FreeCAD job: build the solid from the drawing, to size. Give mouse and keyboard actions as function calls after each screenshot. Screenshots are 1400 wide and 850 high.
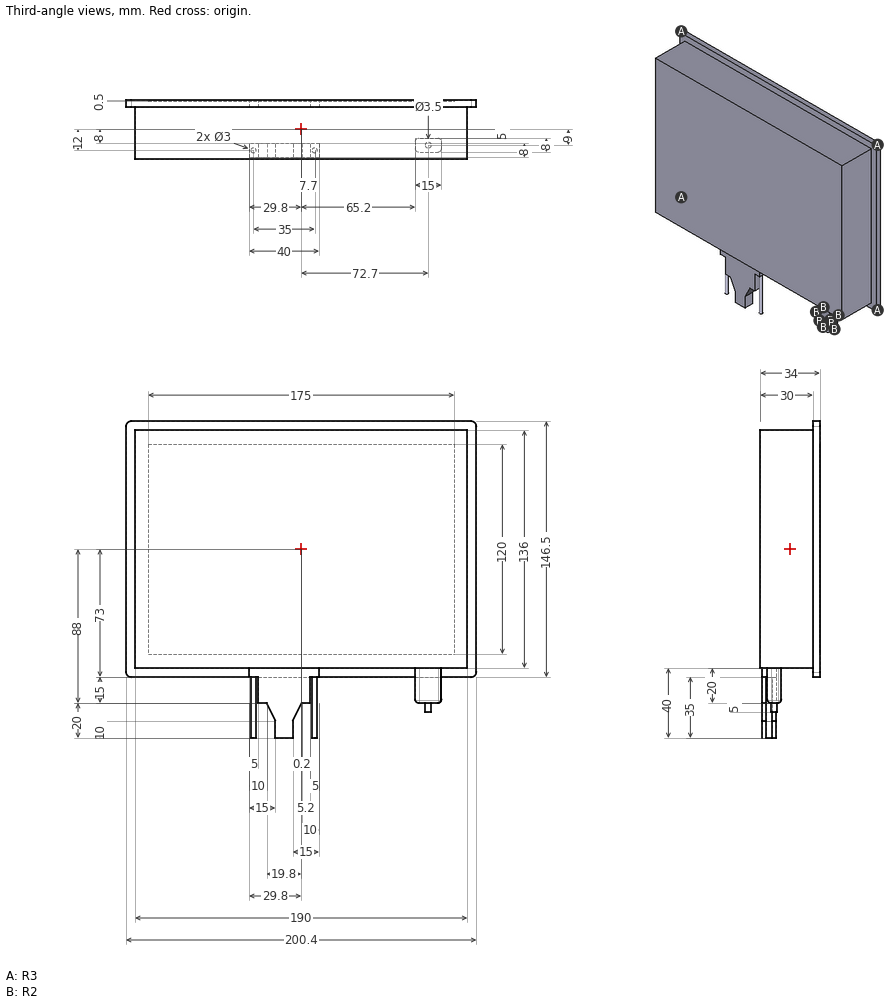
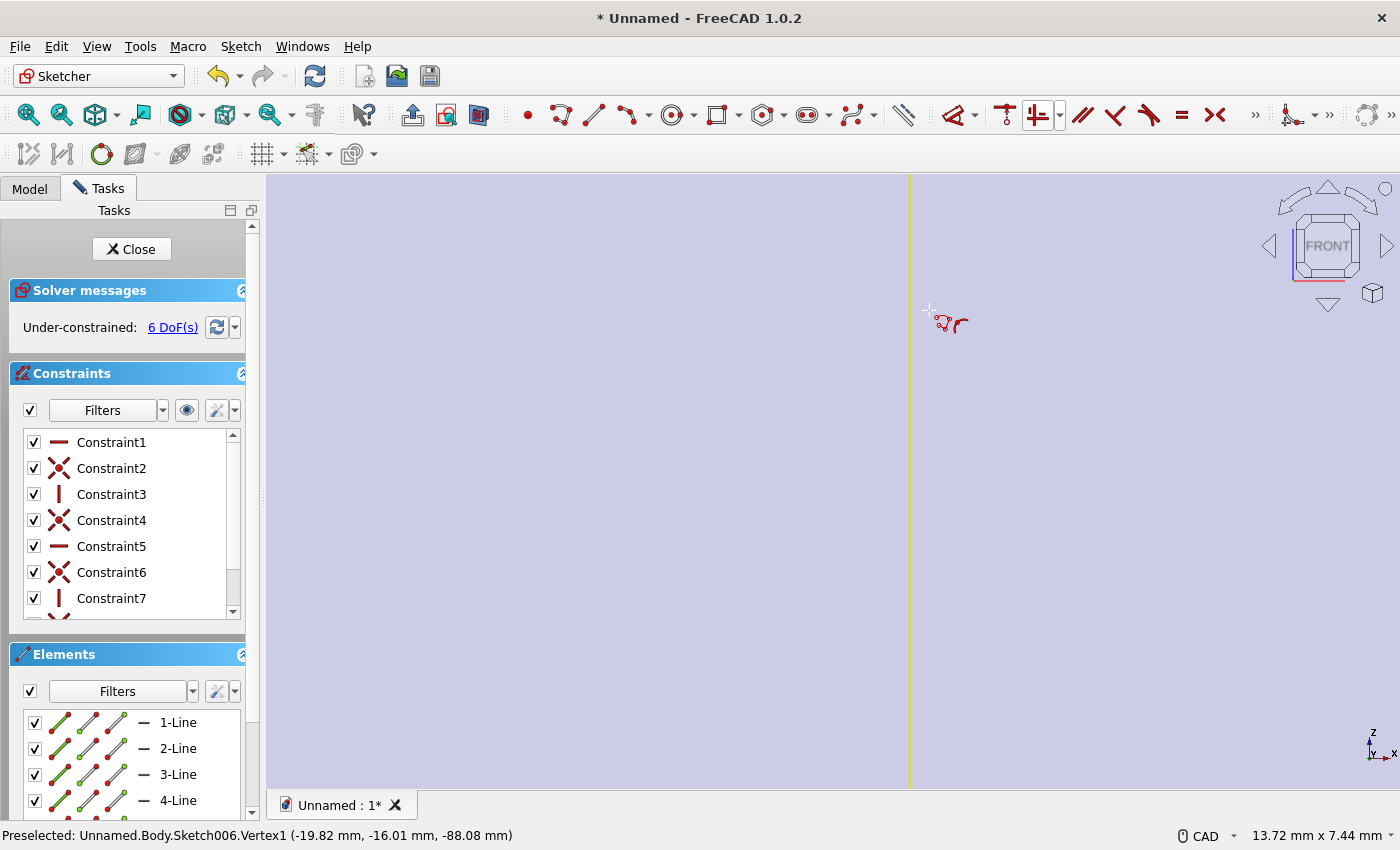
click(927, 308)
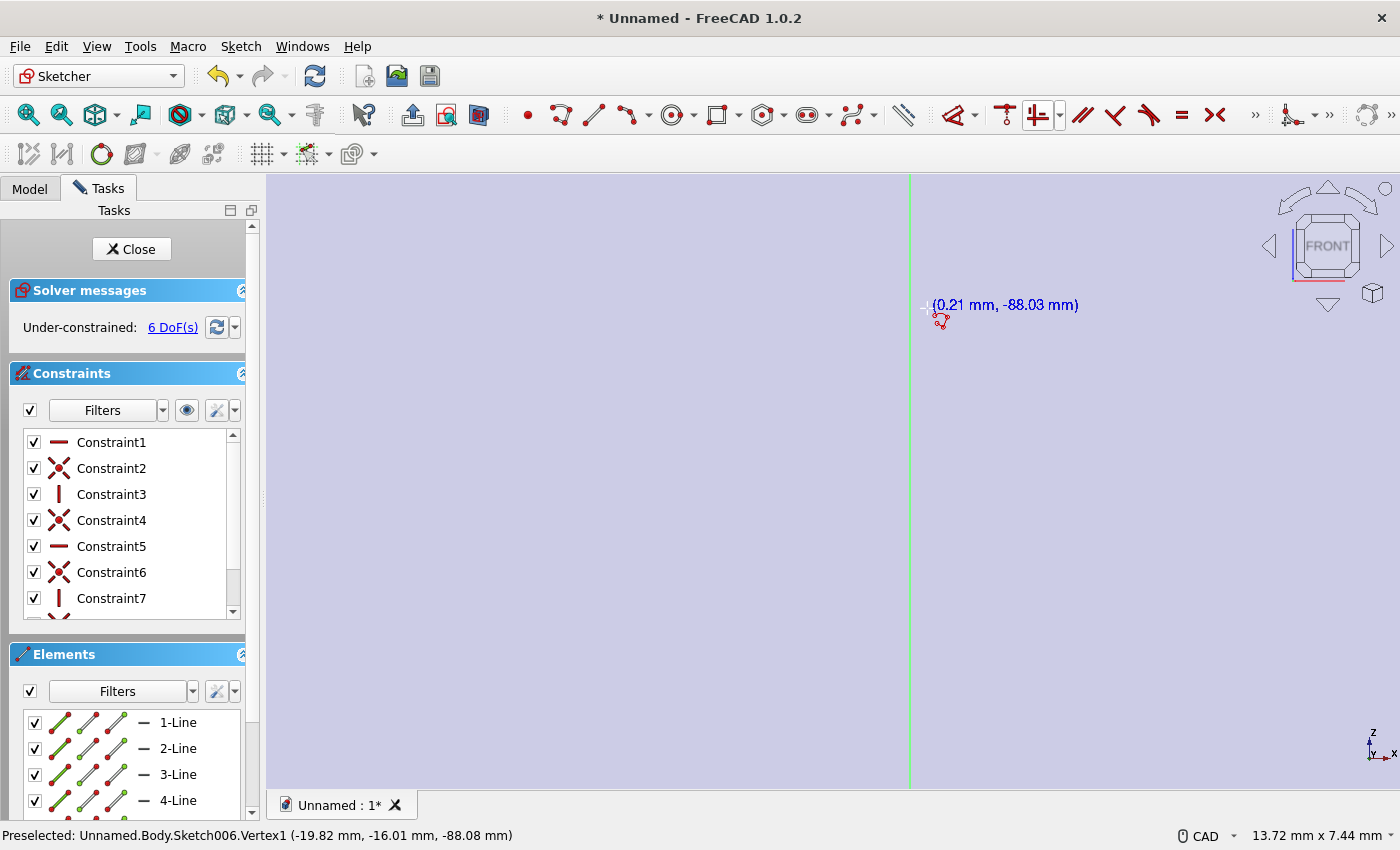
scroll(932, 316, down, 8)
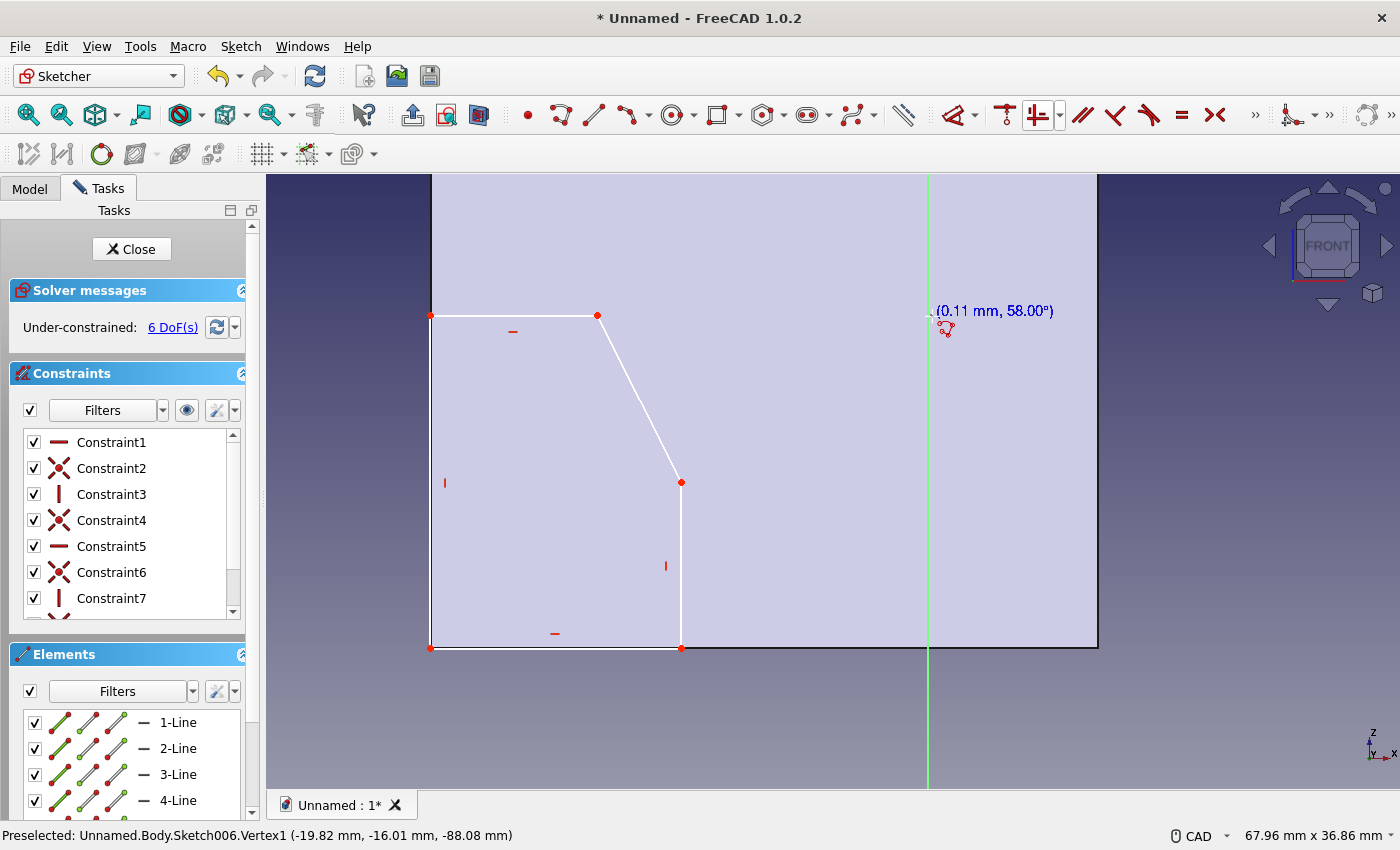
click(848, 481)
click(848, 648)
click(1098, 648)
click(1098, 314)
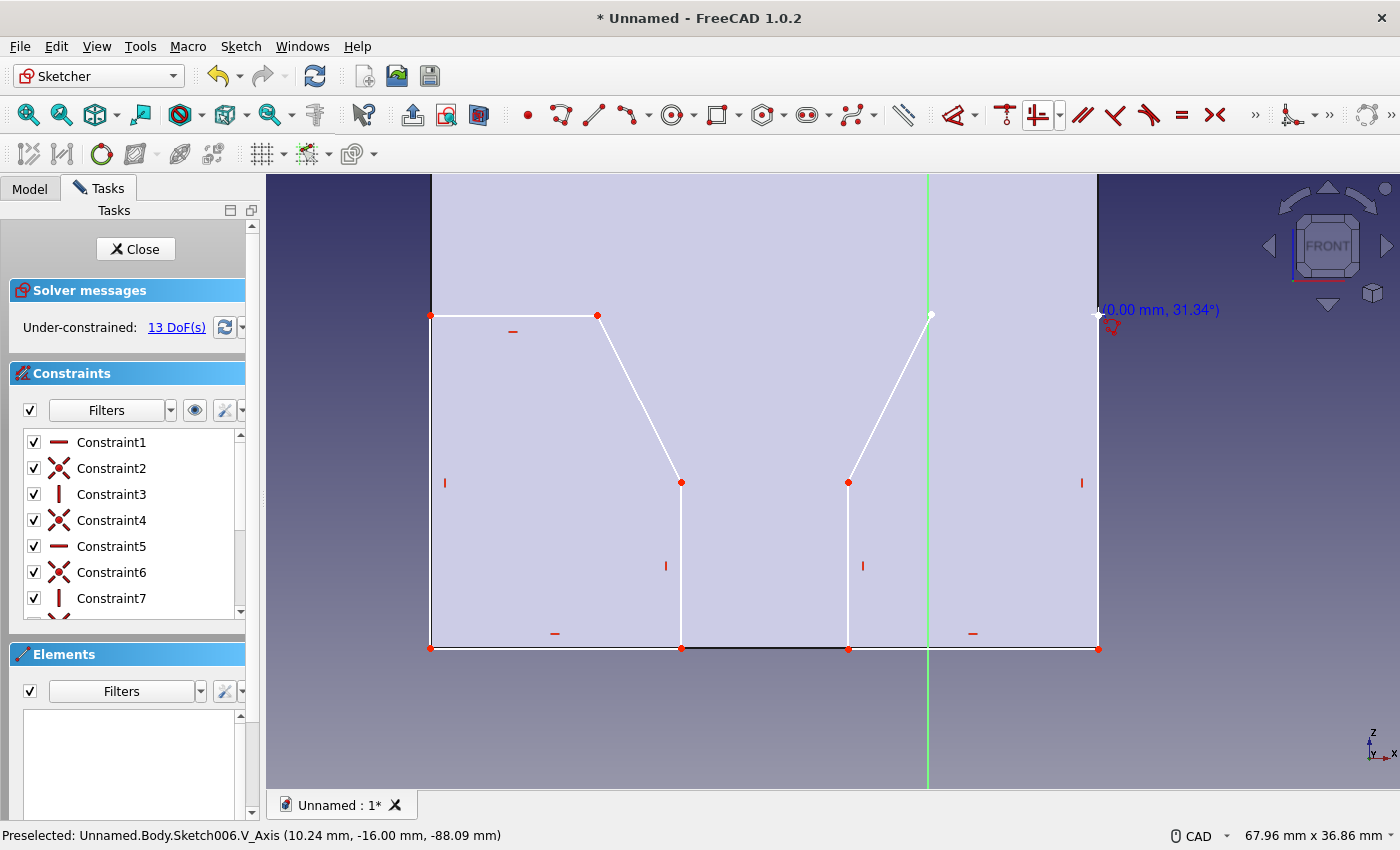
scroll(931, 314, up, 8)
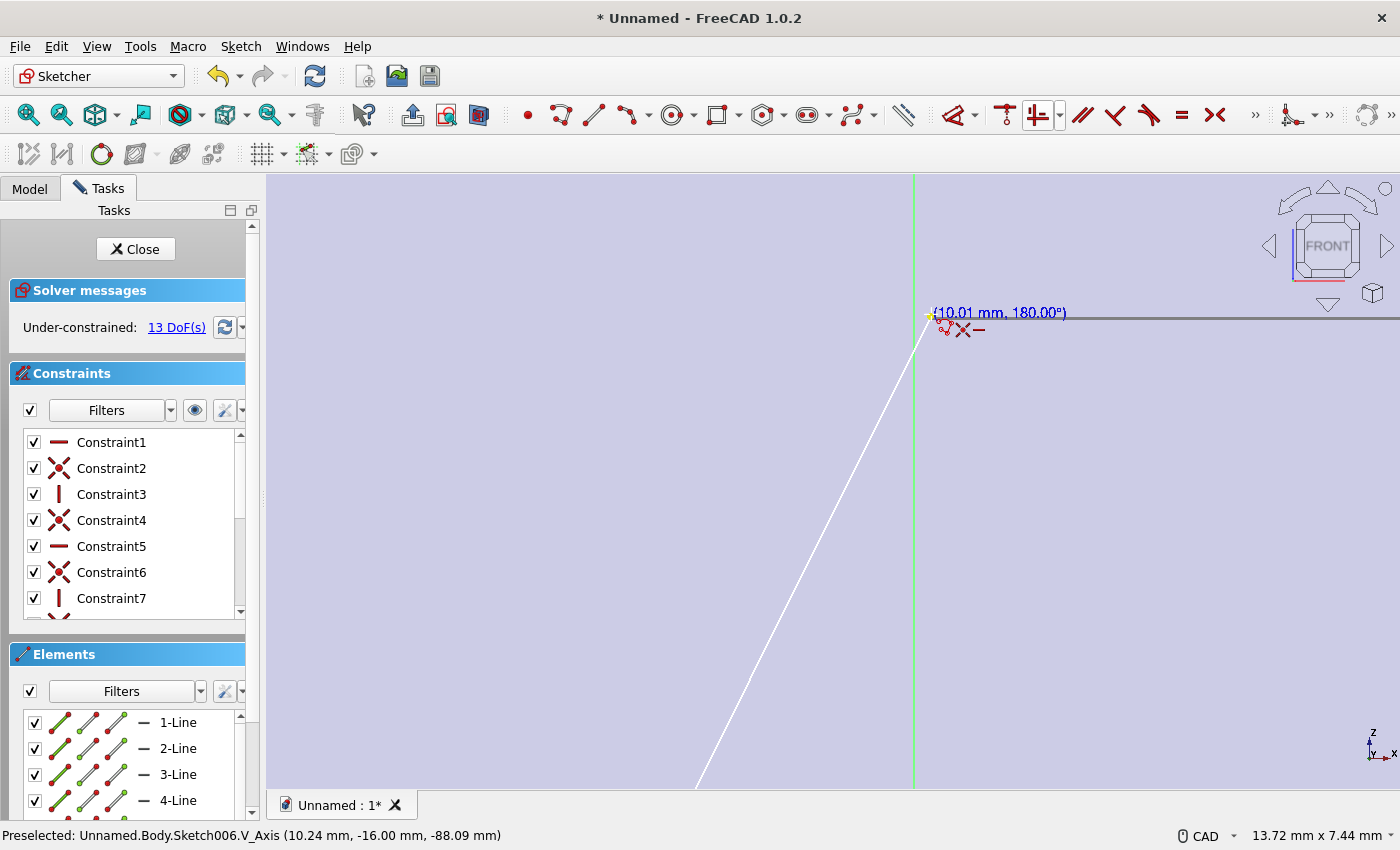
click(931, 317)
key(Escape)
key(Escape)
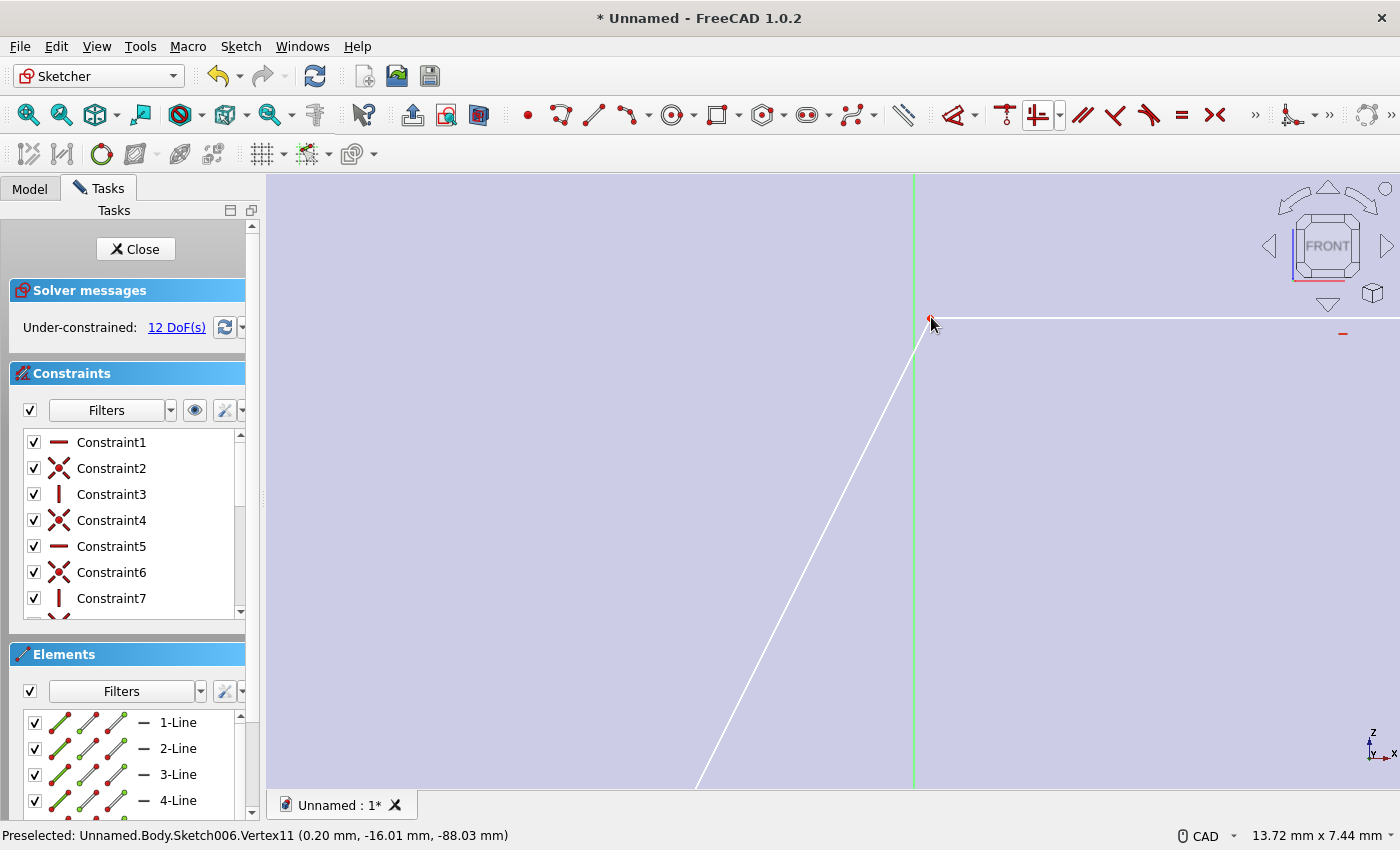
click(952, 116)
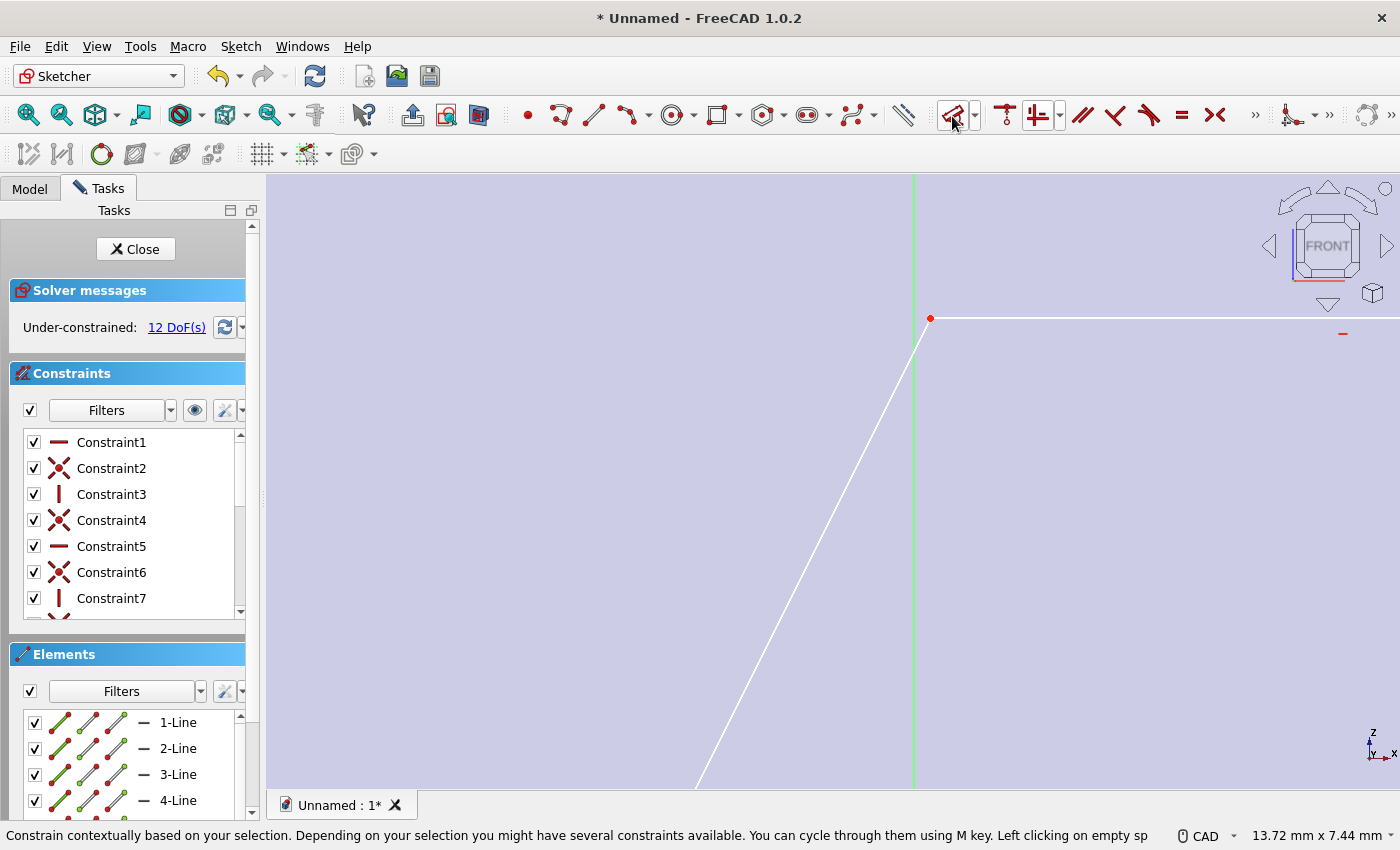
scroll(931, 314, down, 8)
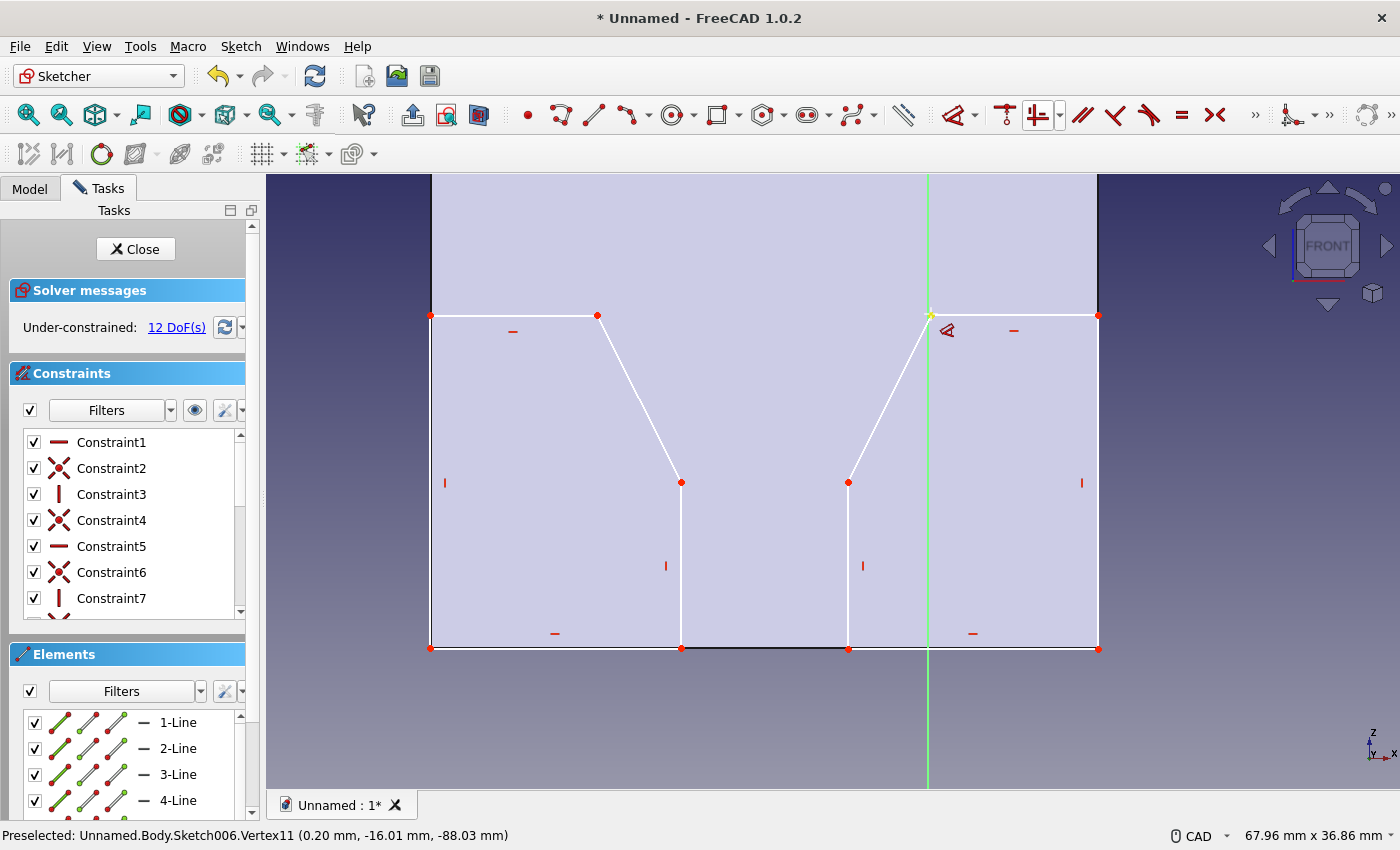
click(547, 316)
click(514, 282)